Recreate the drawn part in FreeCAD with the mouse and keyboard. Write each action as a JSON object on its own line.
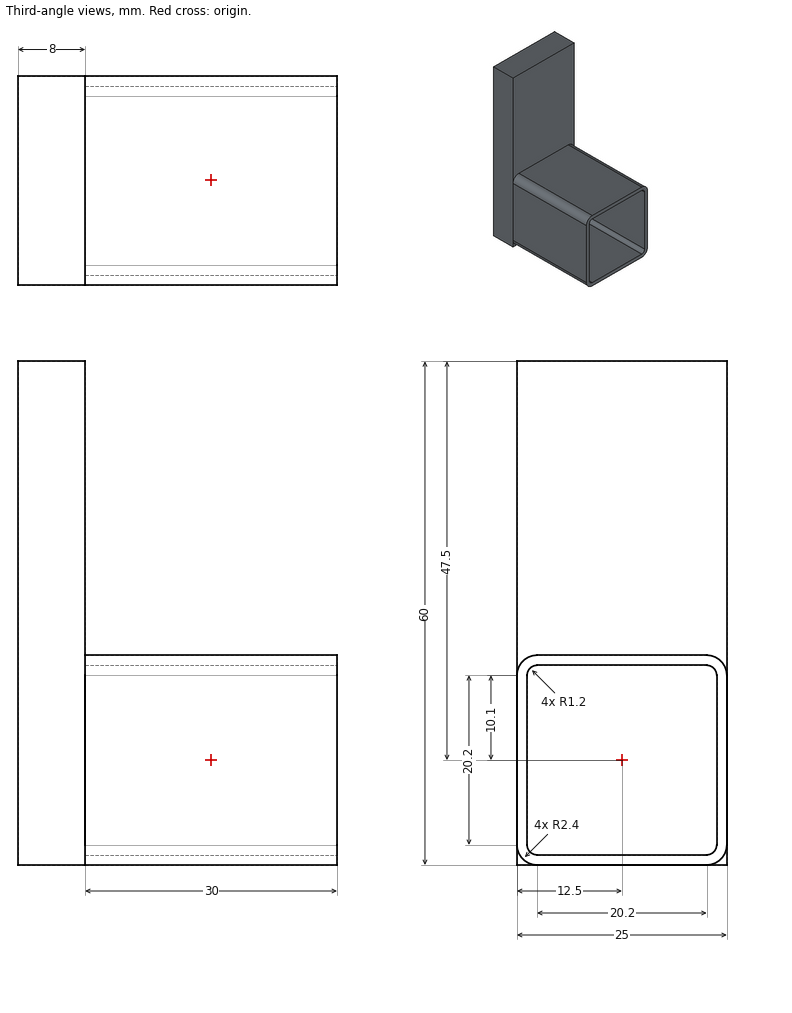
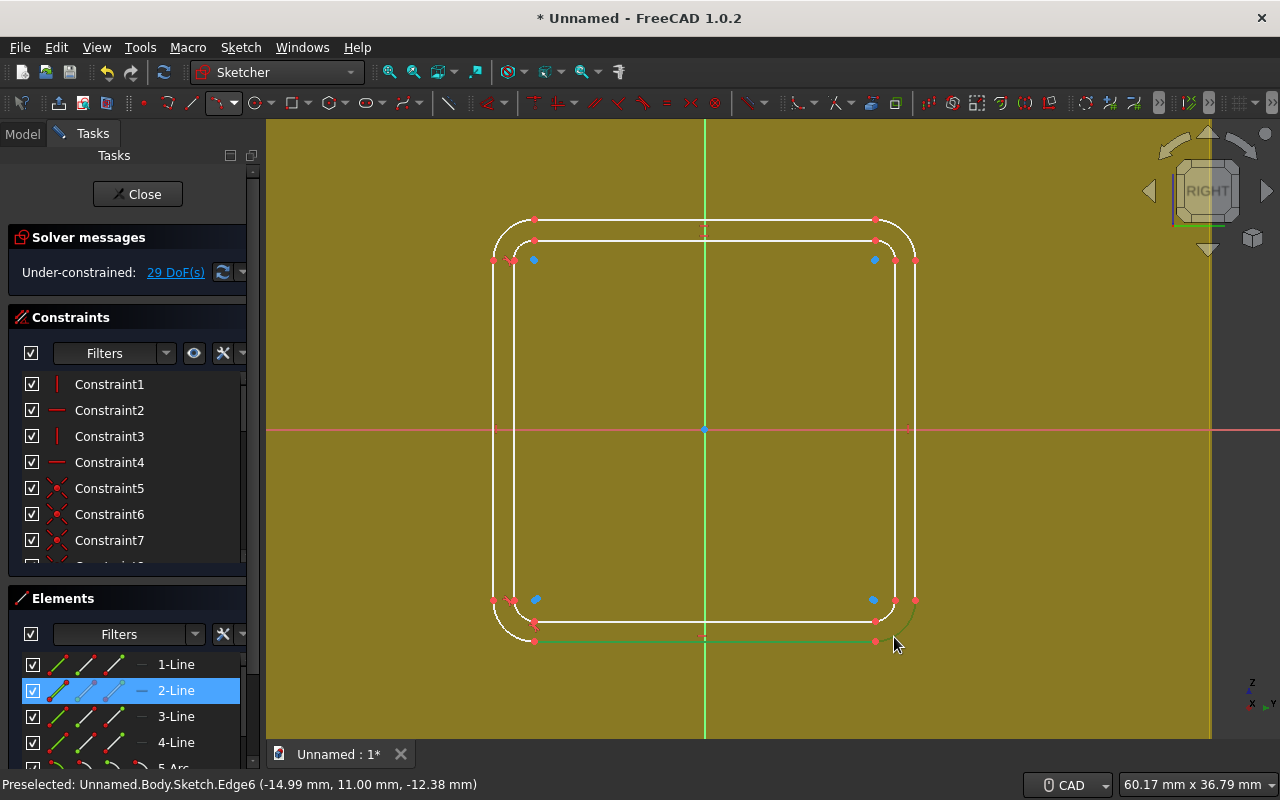
{"action": "key", "text": "t"}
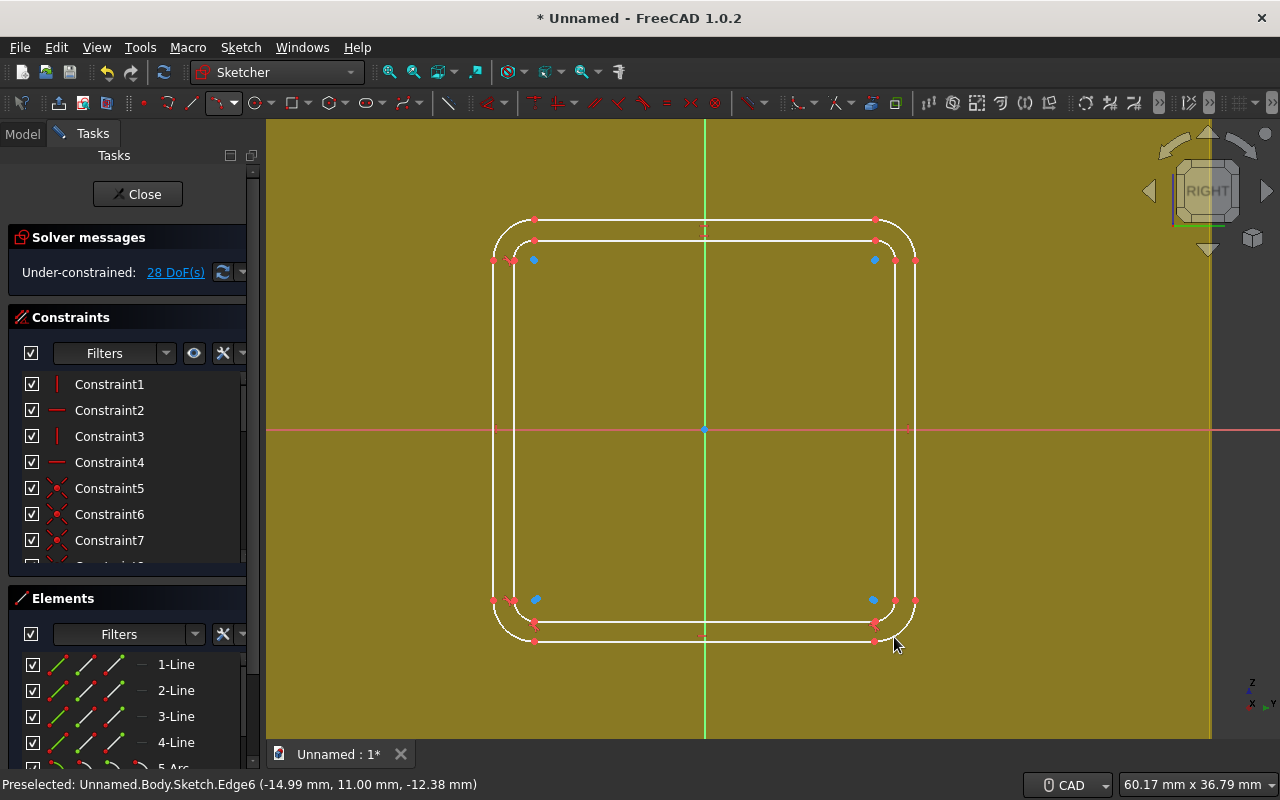
{"action": "left_click", "coordinate": [915, 499]}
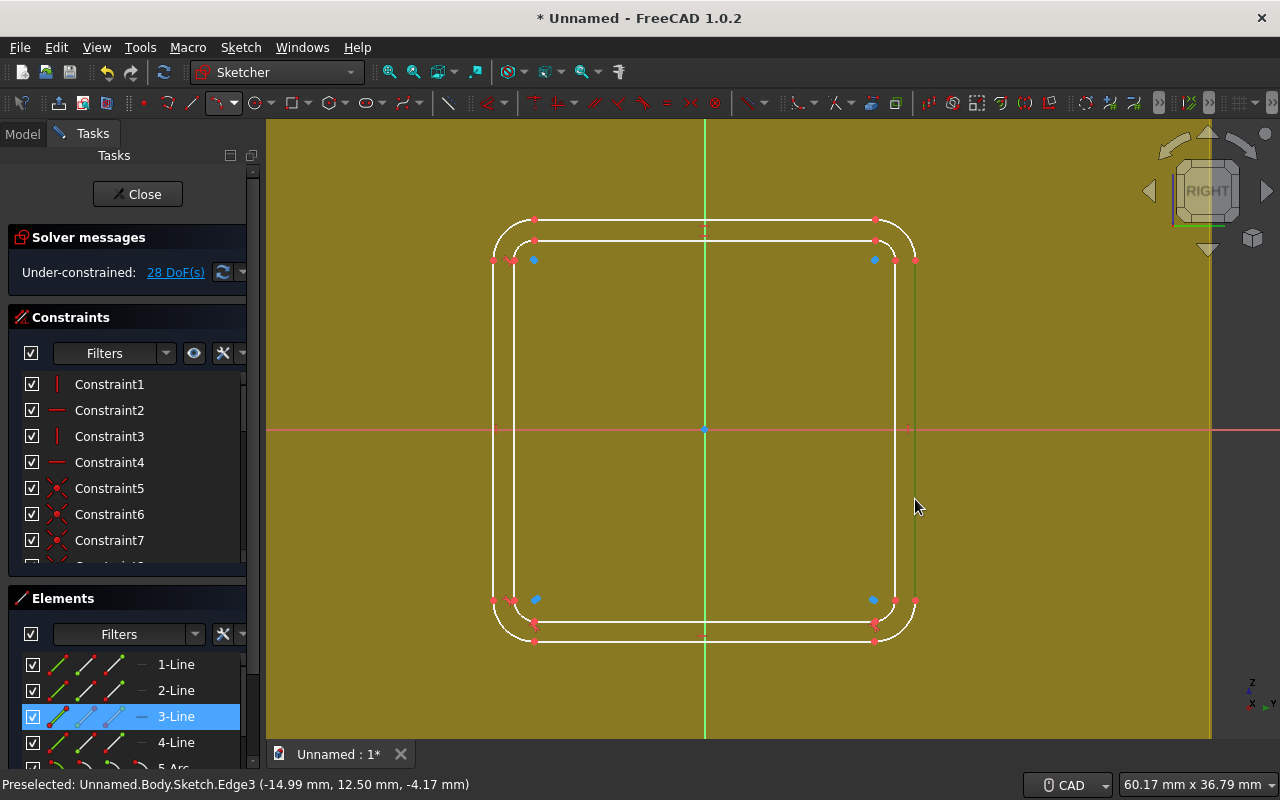
{"action": "left_click", "coordinate": [893, 637]}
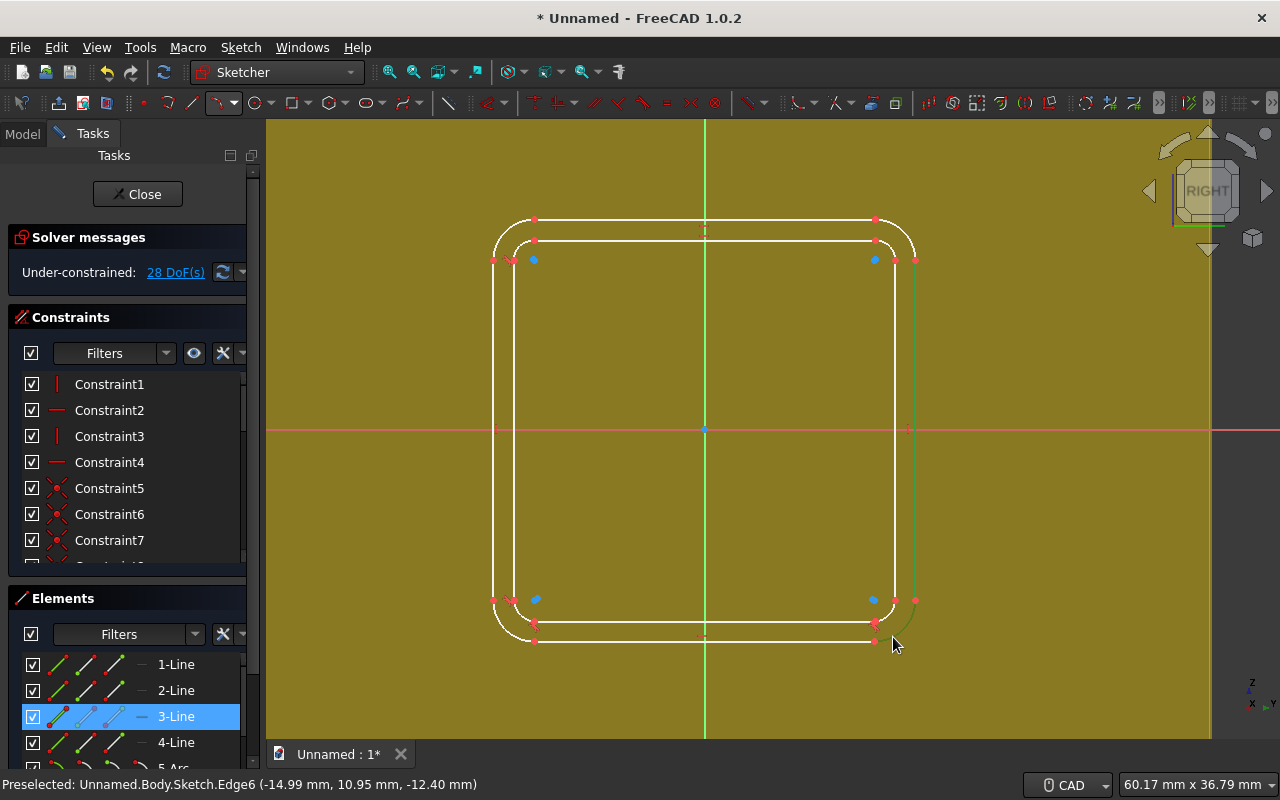
{"action": "key", "text": "t"}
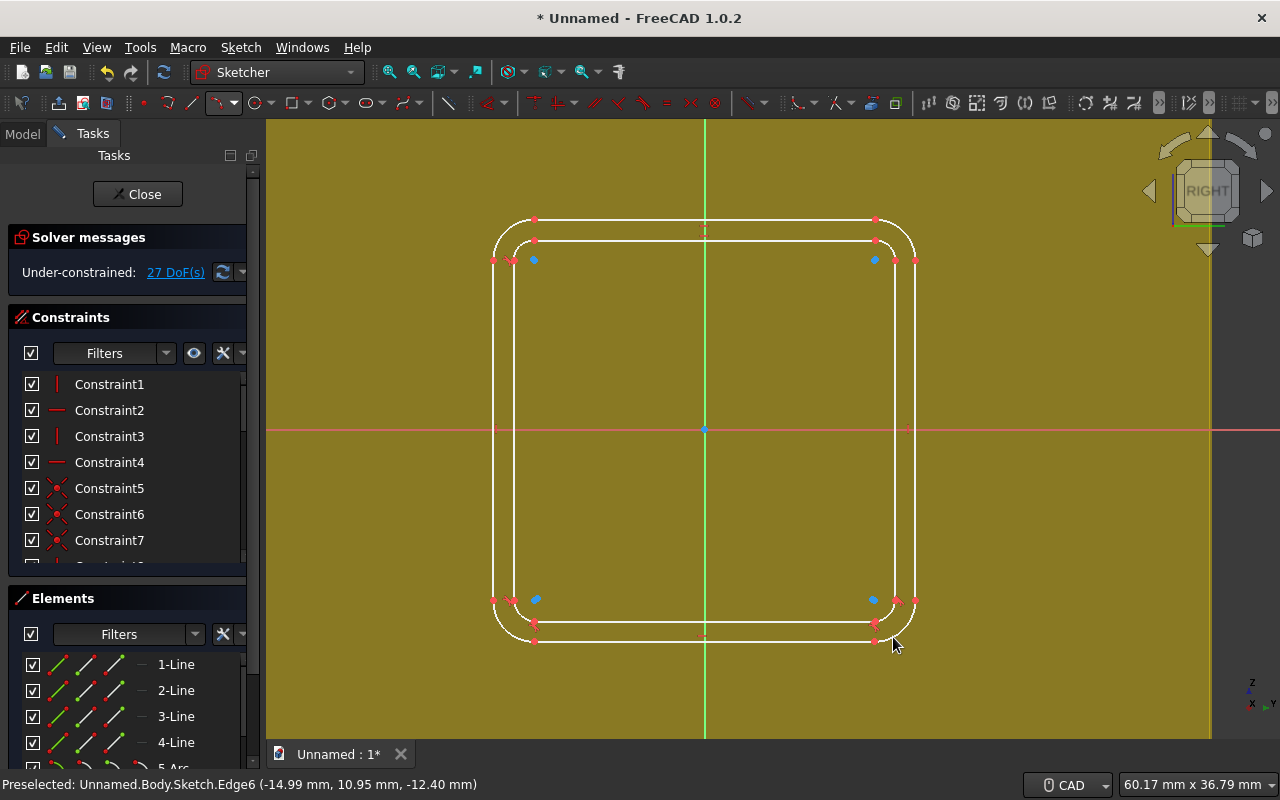
{"action": "left_click", "coordinate": [915, 499]}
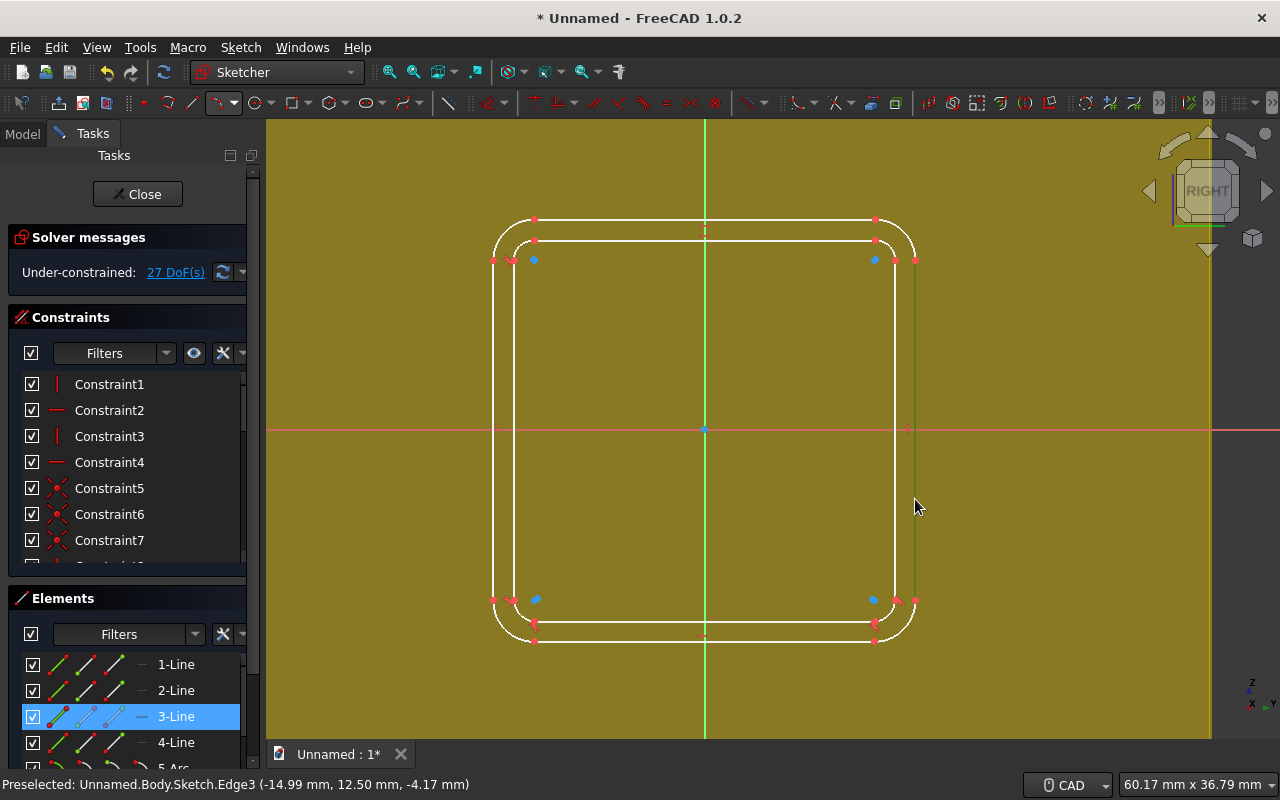
{"action": "left_click", "coordinate": [911, 242]}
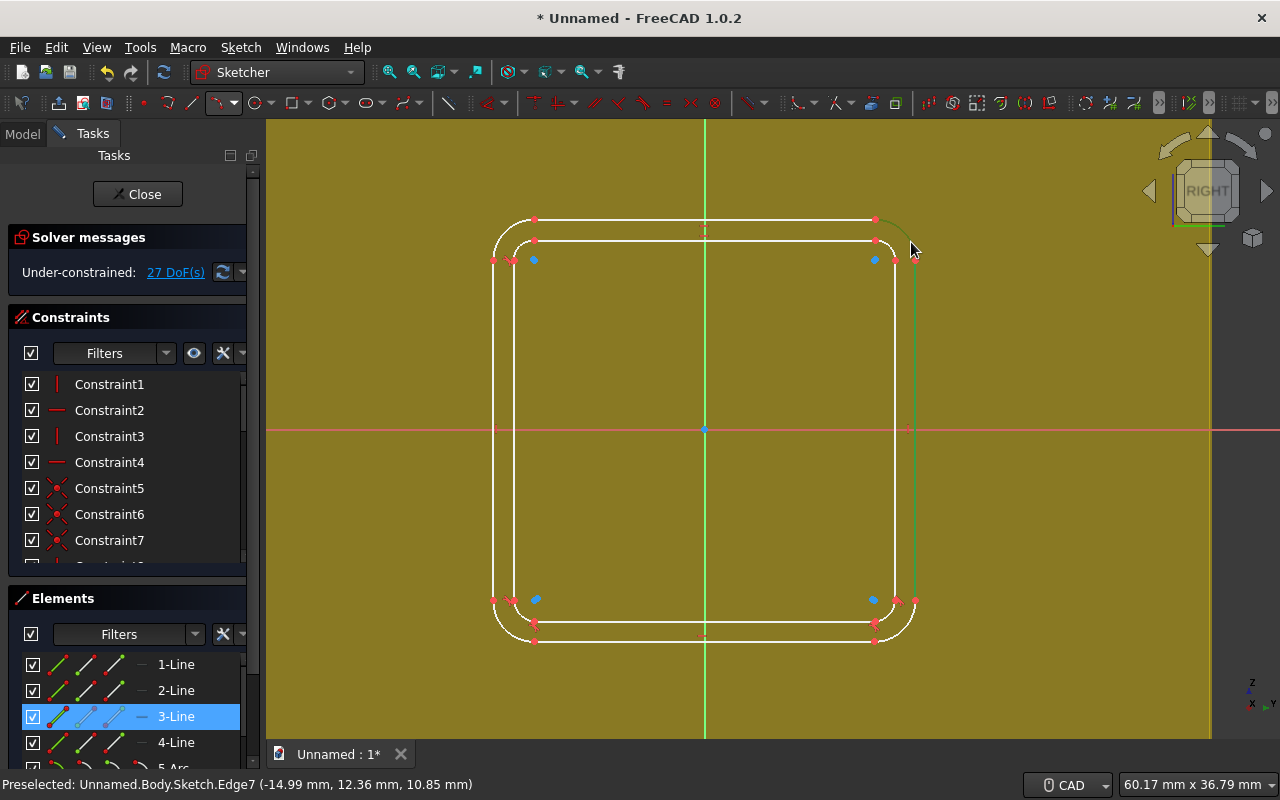
{"action": "key", "text": "t"}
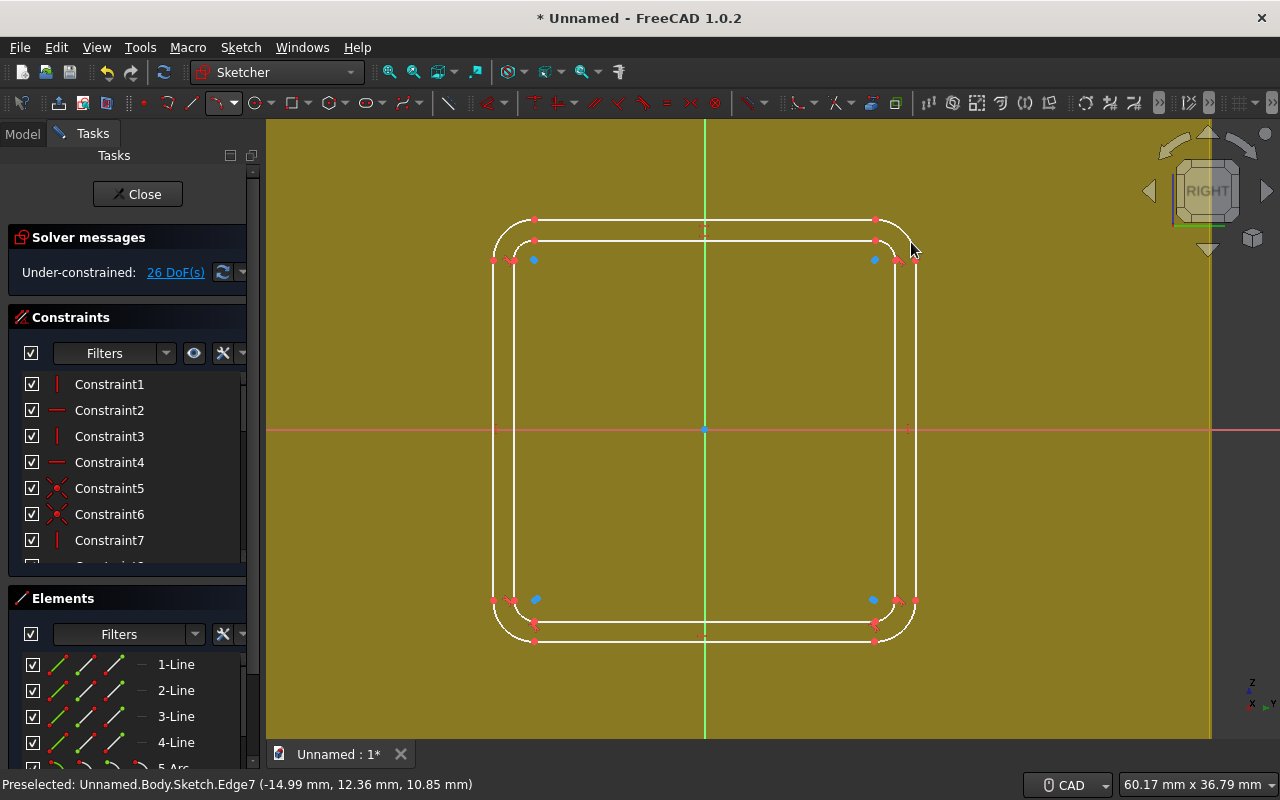
{"action": "left_click", "coordinate": [773, 220]}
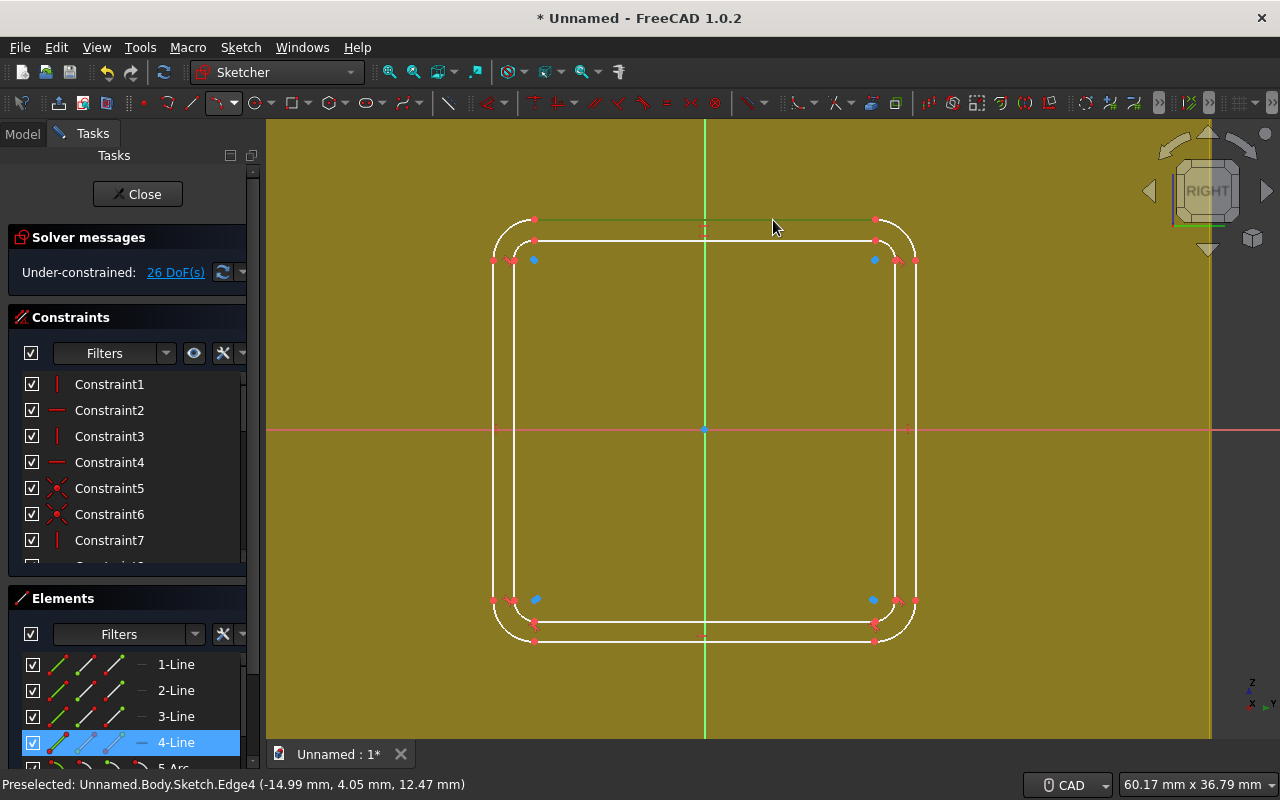
{"action": "left_click", "coordinate": [911, 242]}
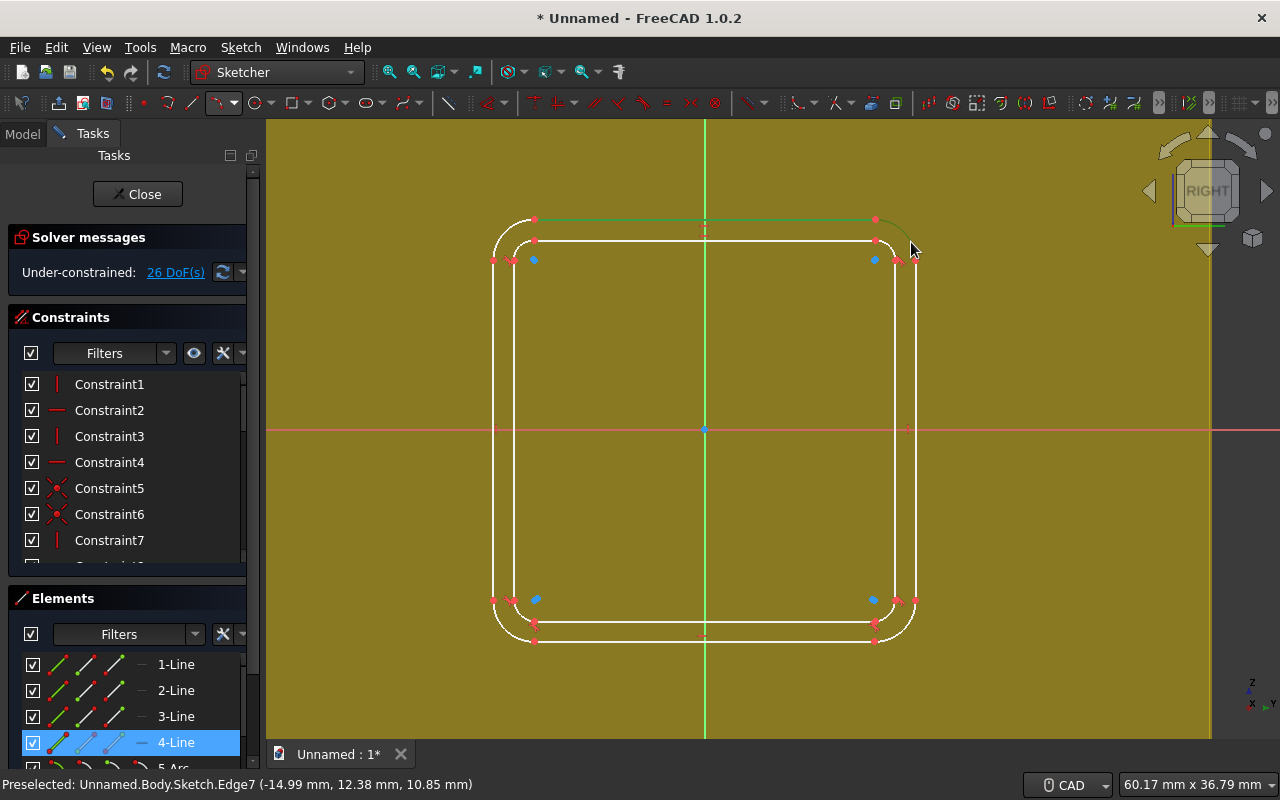
{"action": "key", "text": "t"}